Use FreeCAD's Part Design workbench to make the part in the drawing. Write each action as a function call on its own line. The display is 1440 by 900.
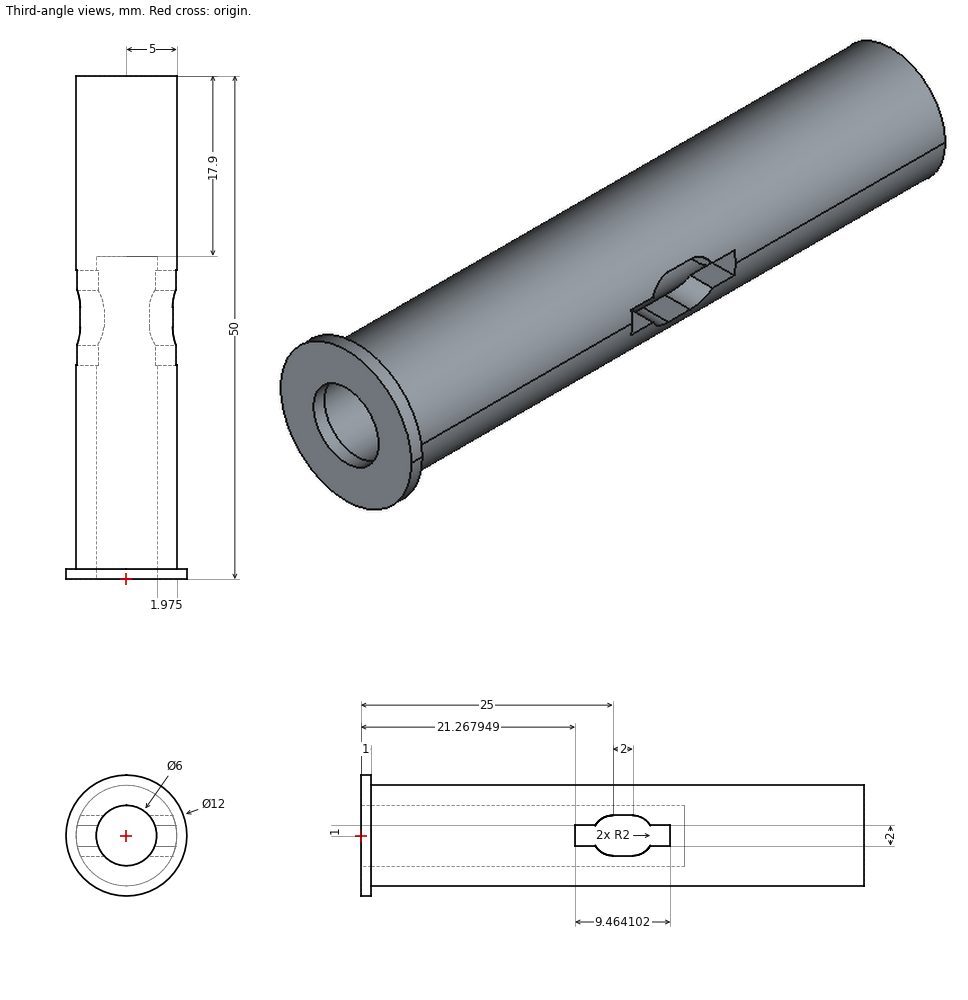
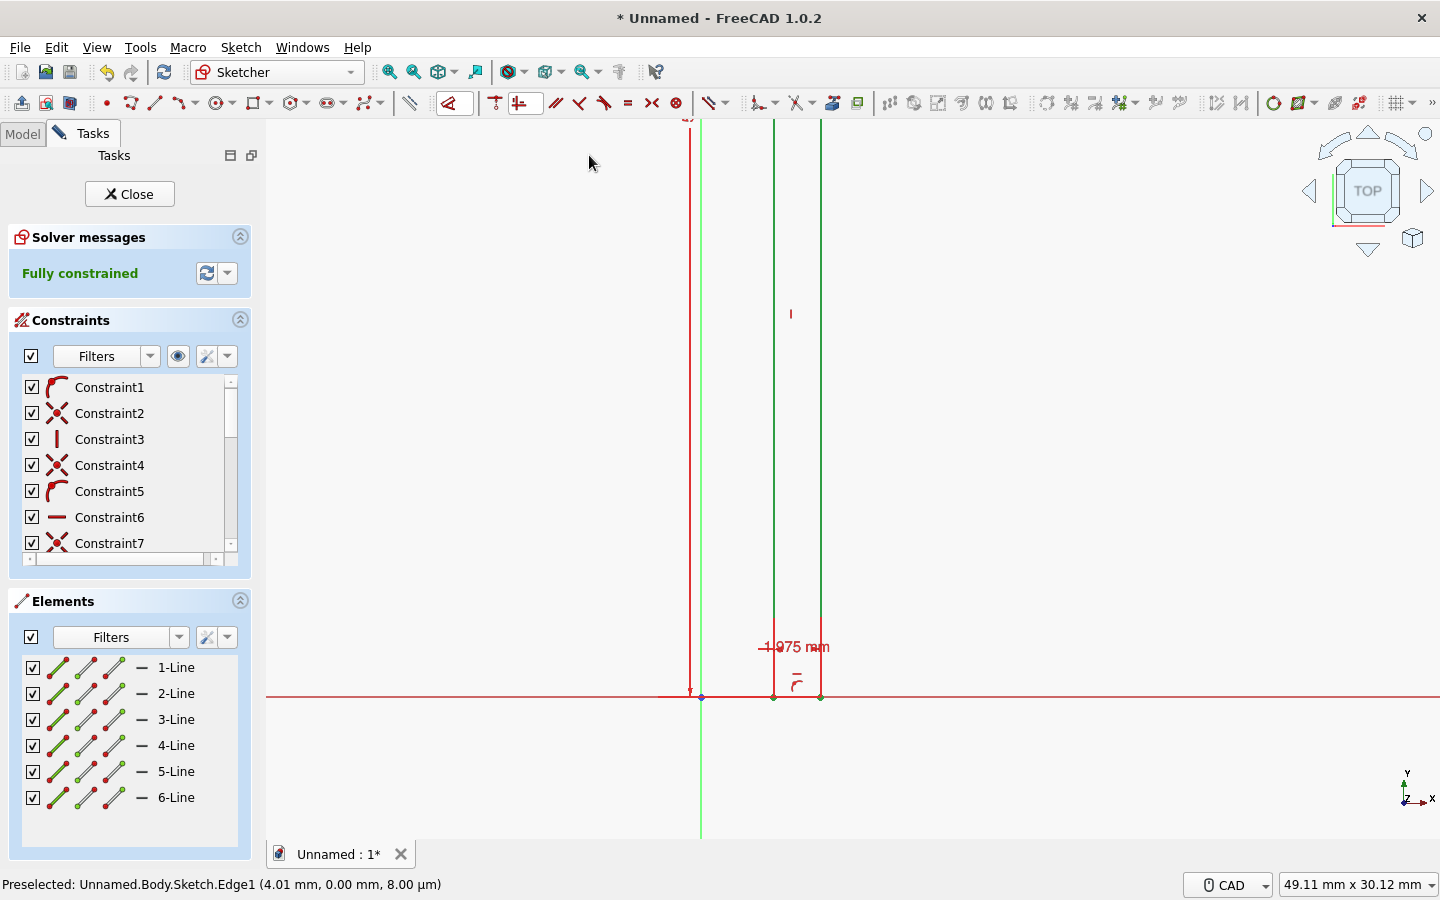
click(130, 194)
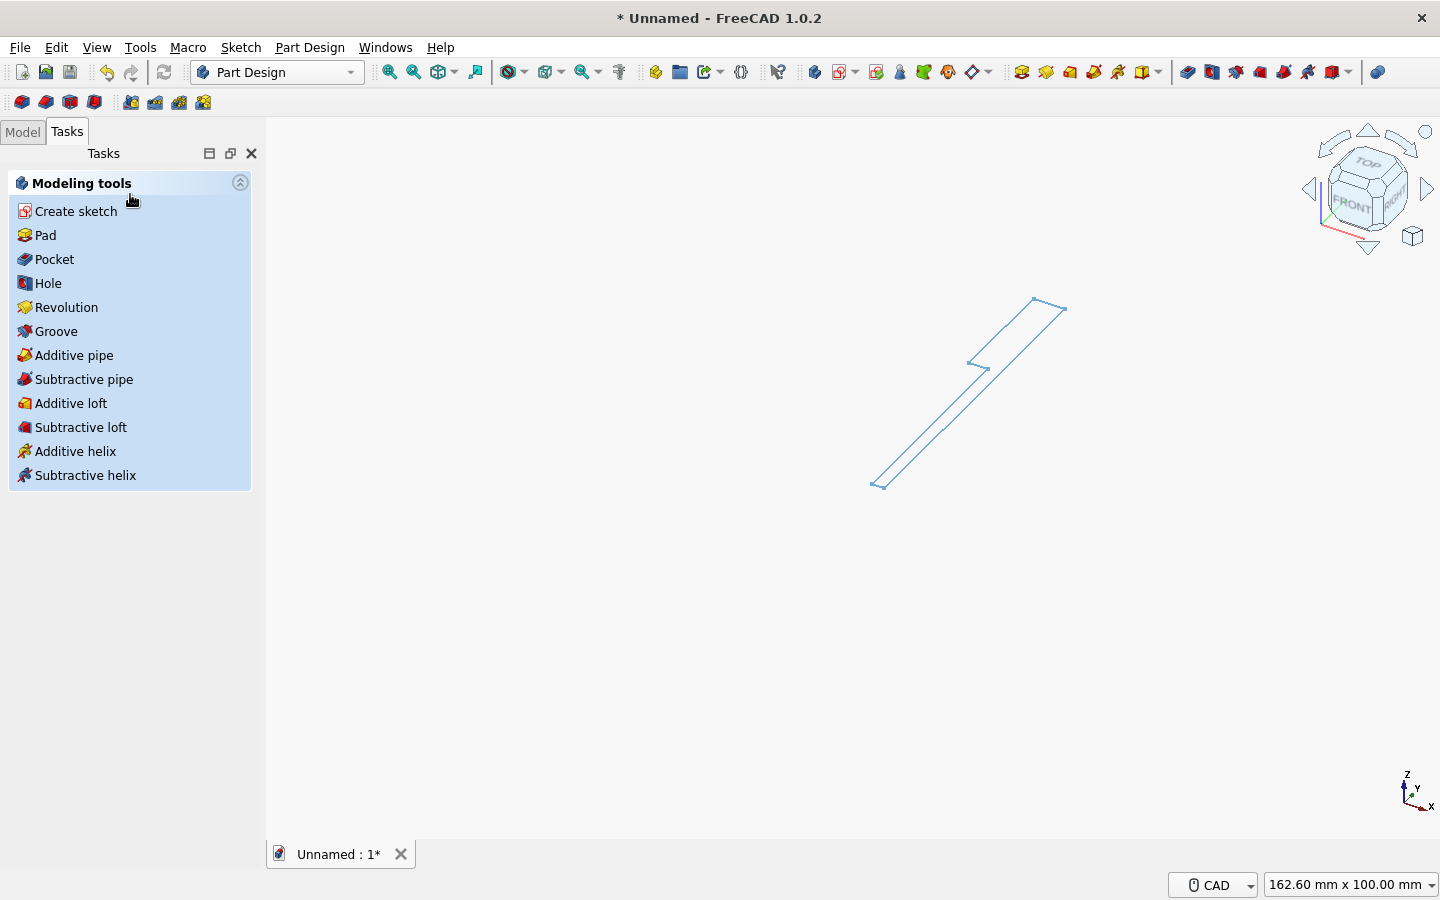
click(1046, 72)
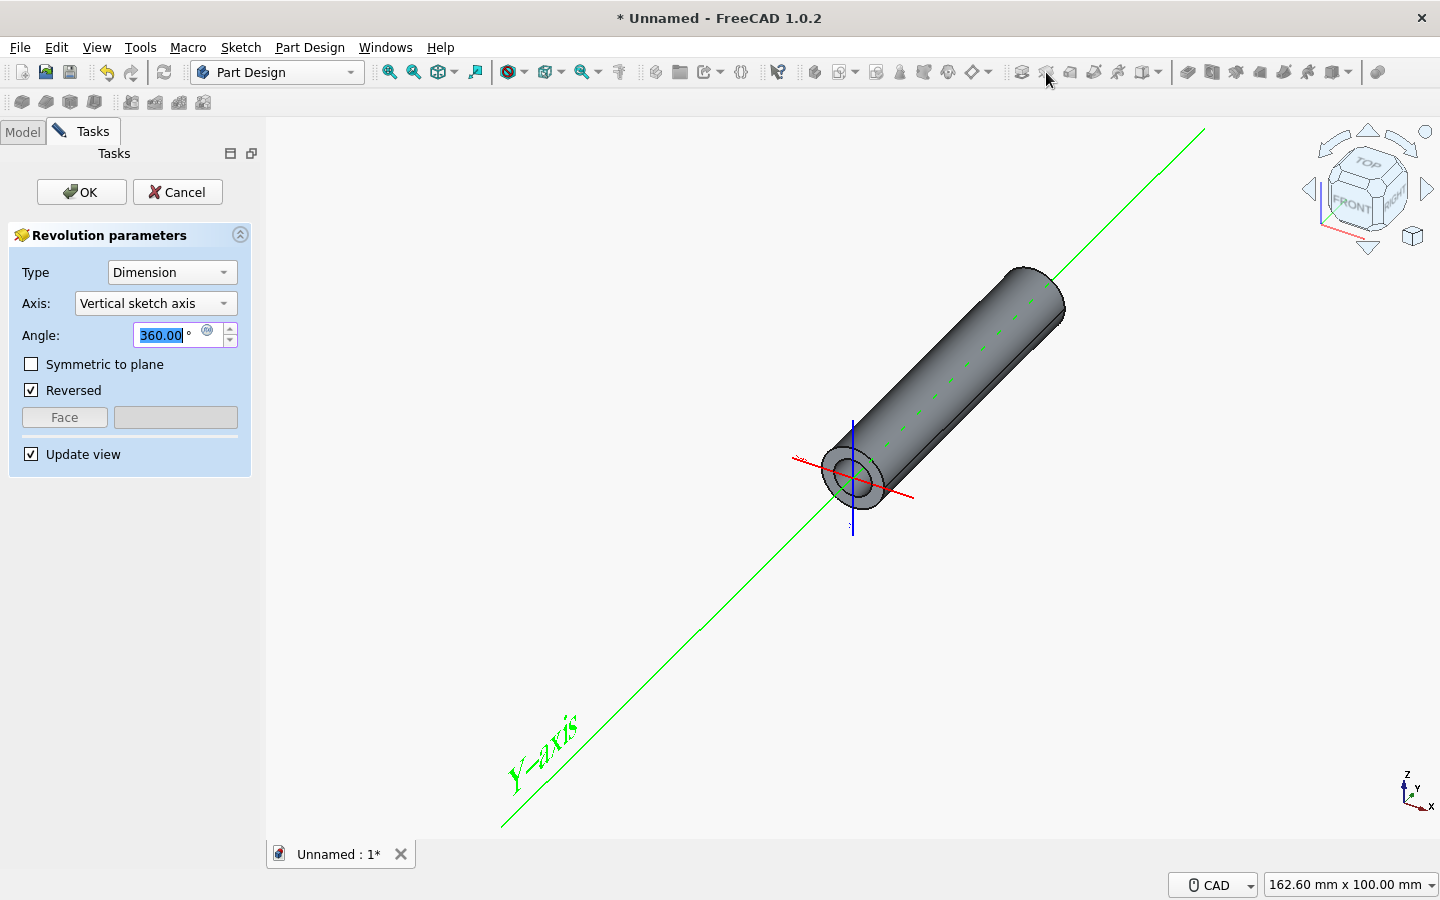
click(82, 192)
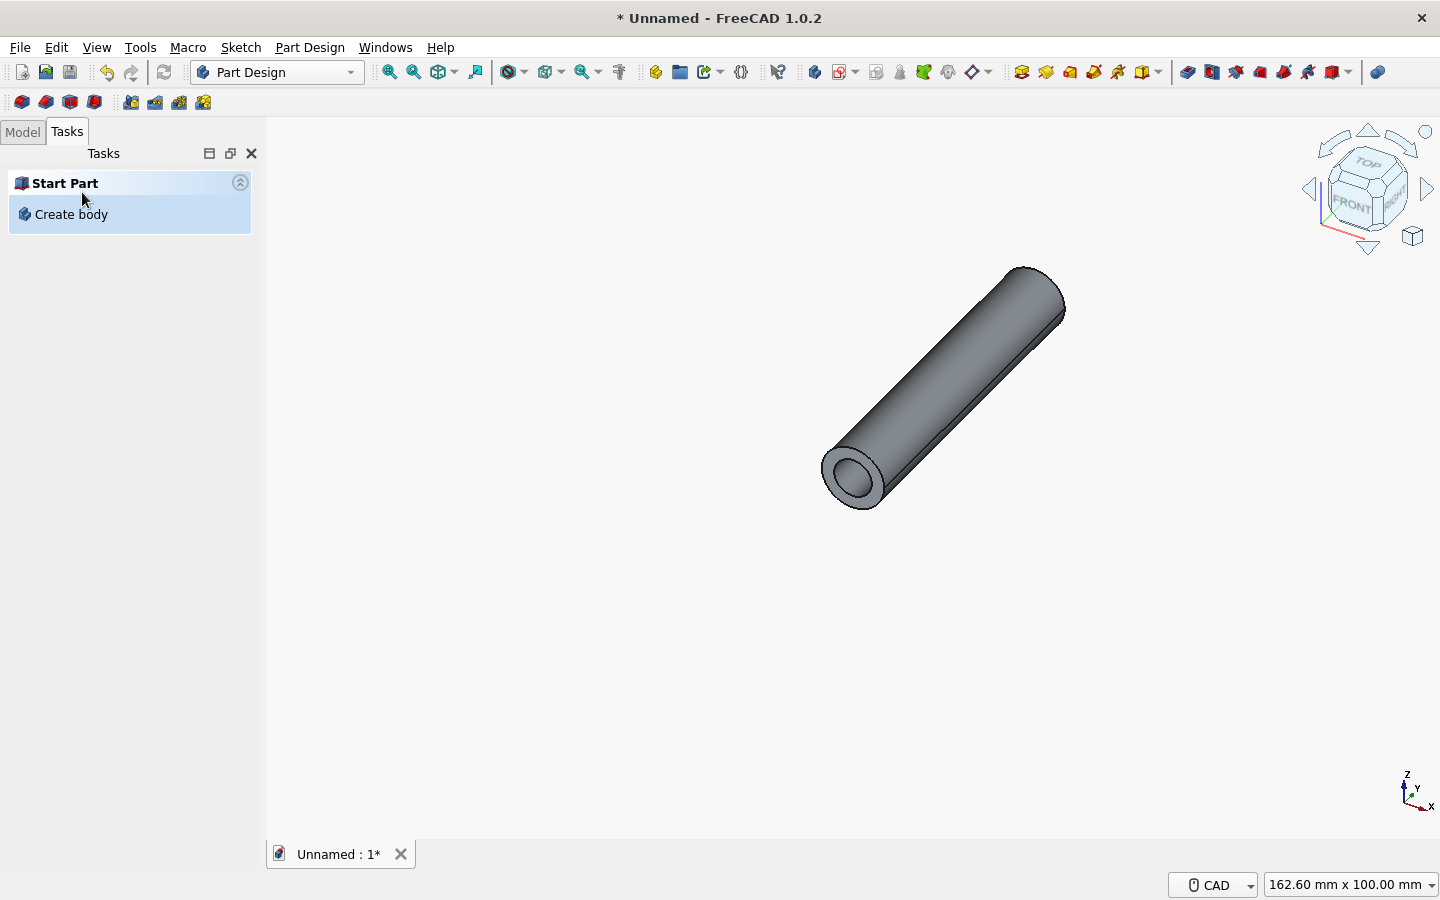
key(v)
key(f)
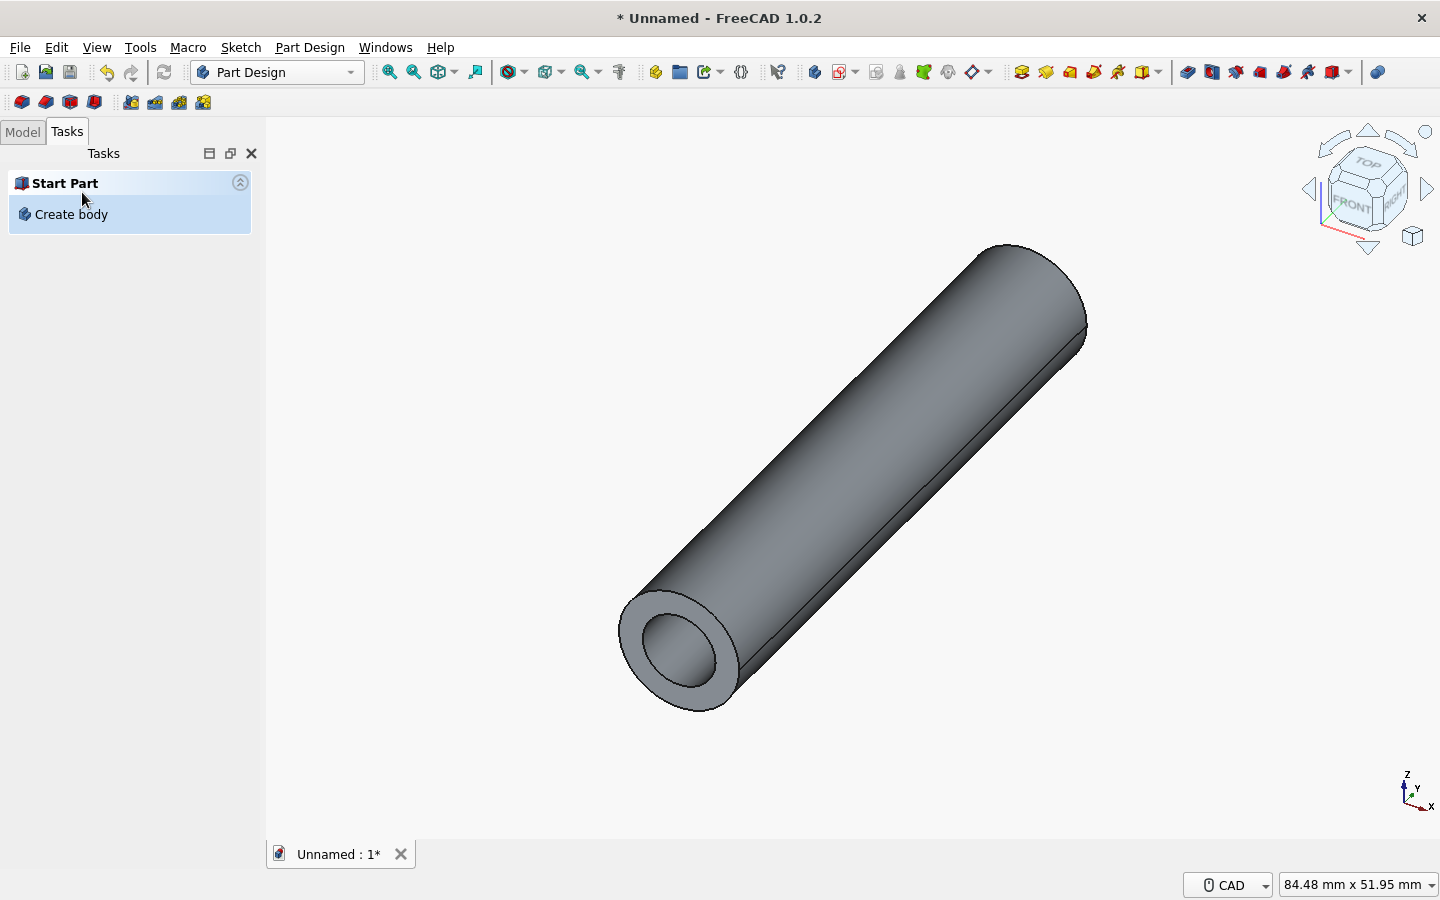
click(23, 131)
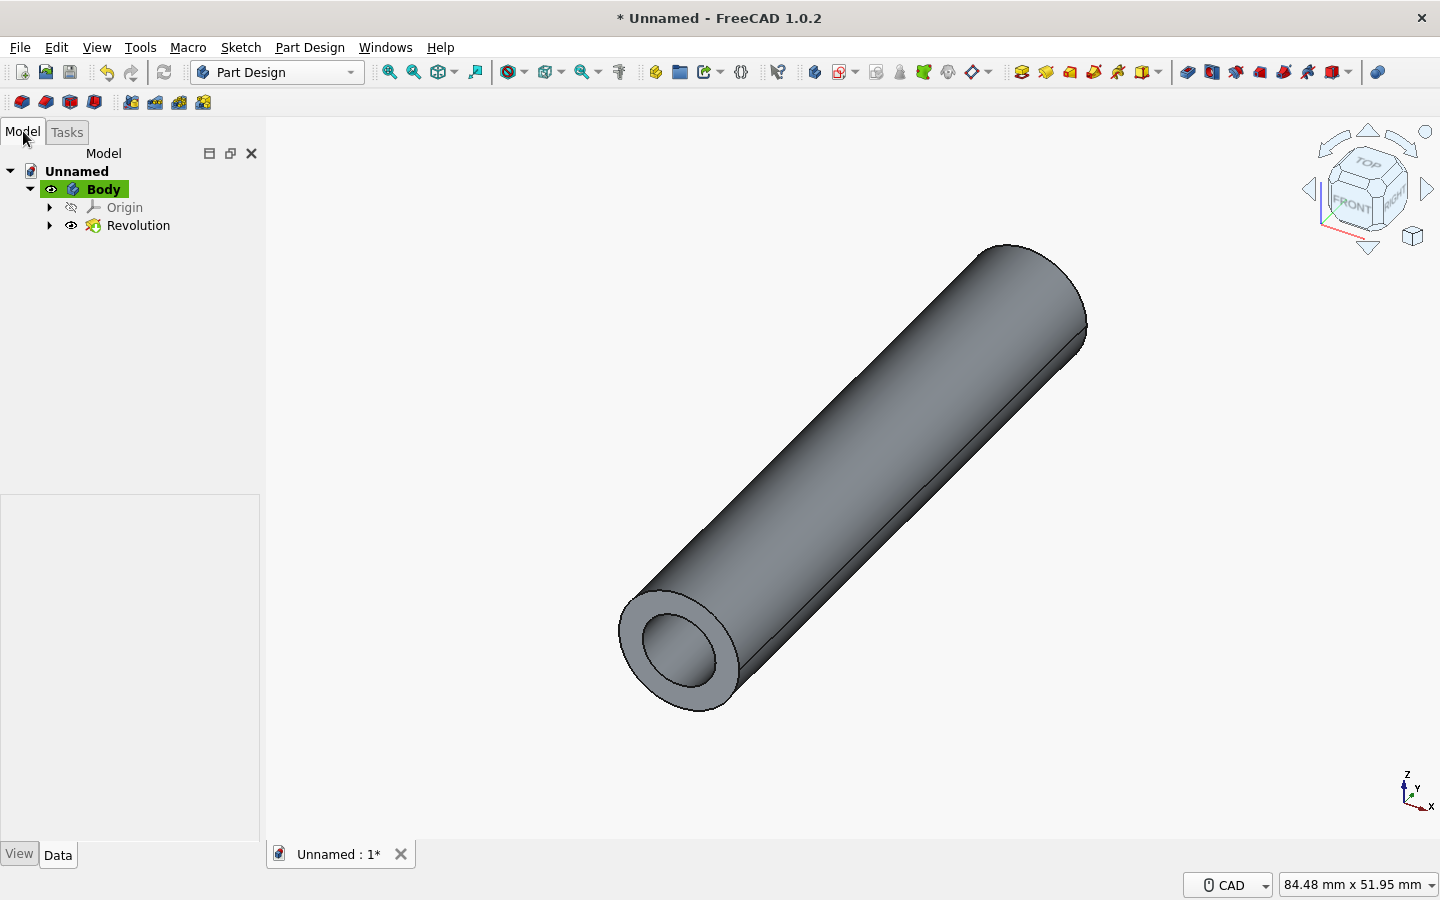
click(50, 207)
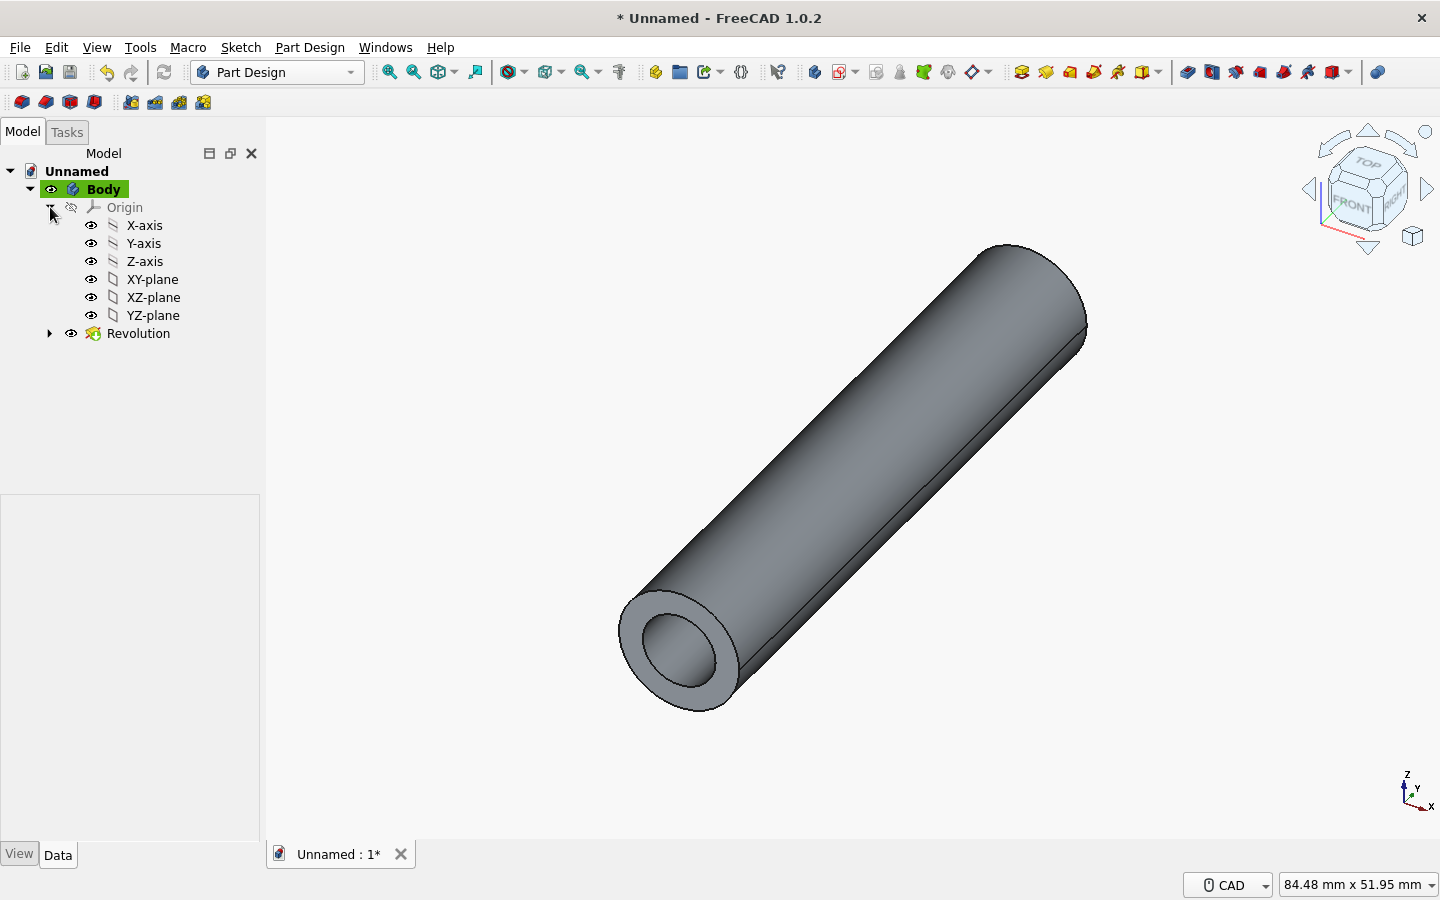
click(136, 315)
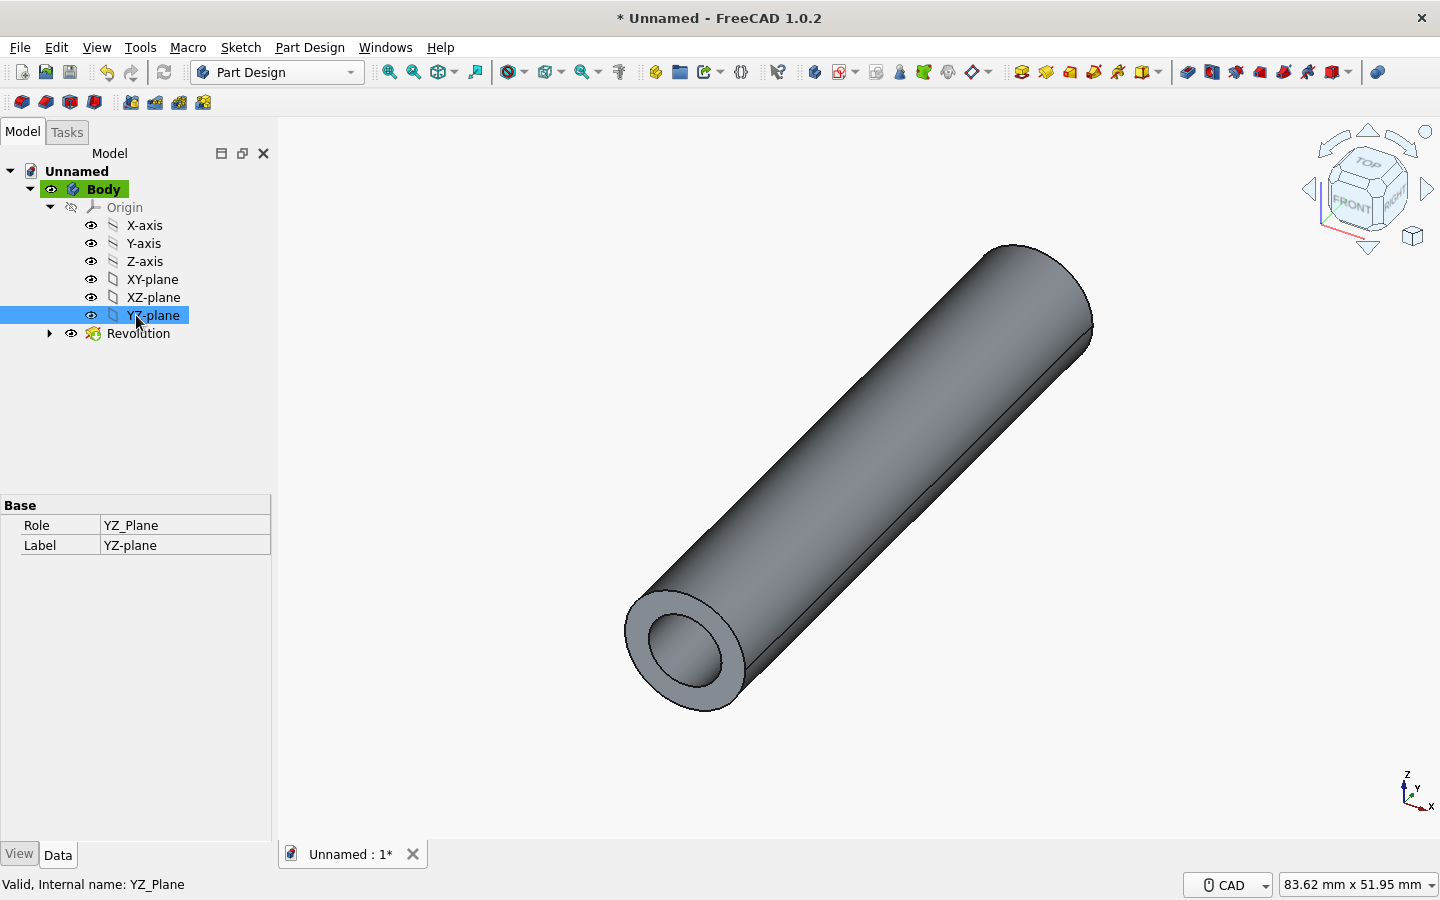
click(972, 72)